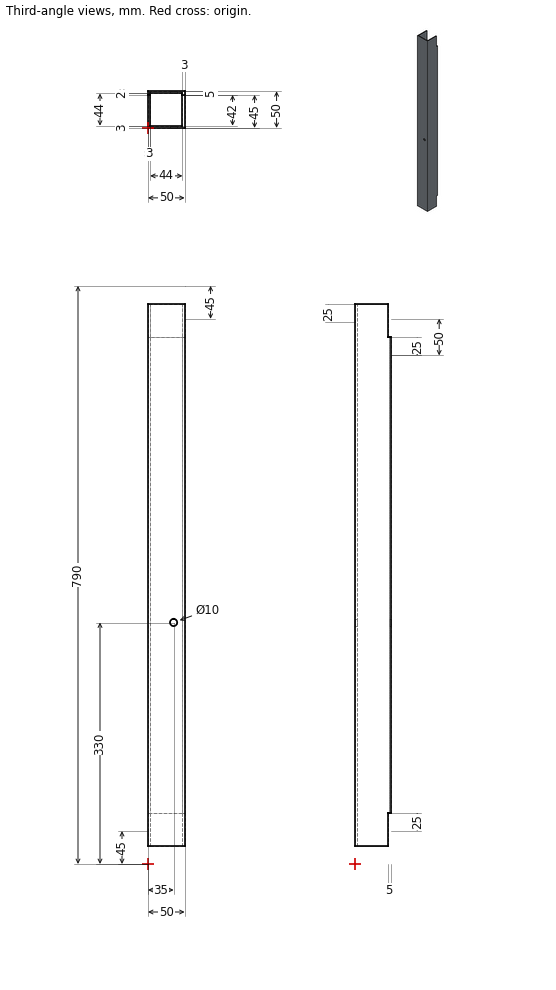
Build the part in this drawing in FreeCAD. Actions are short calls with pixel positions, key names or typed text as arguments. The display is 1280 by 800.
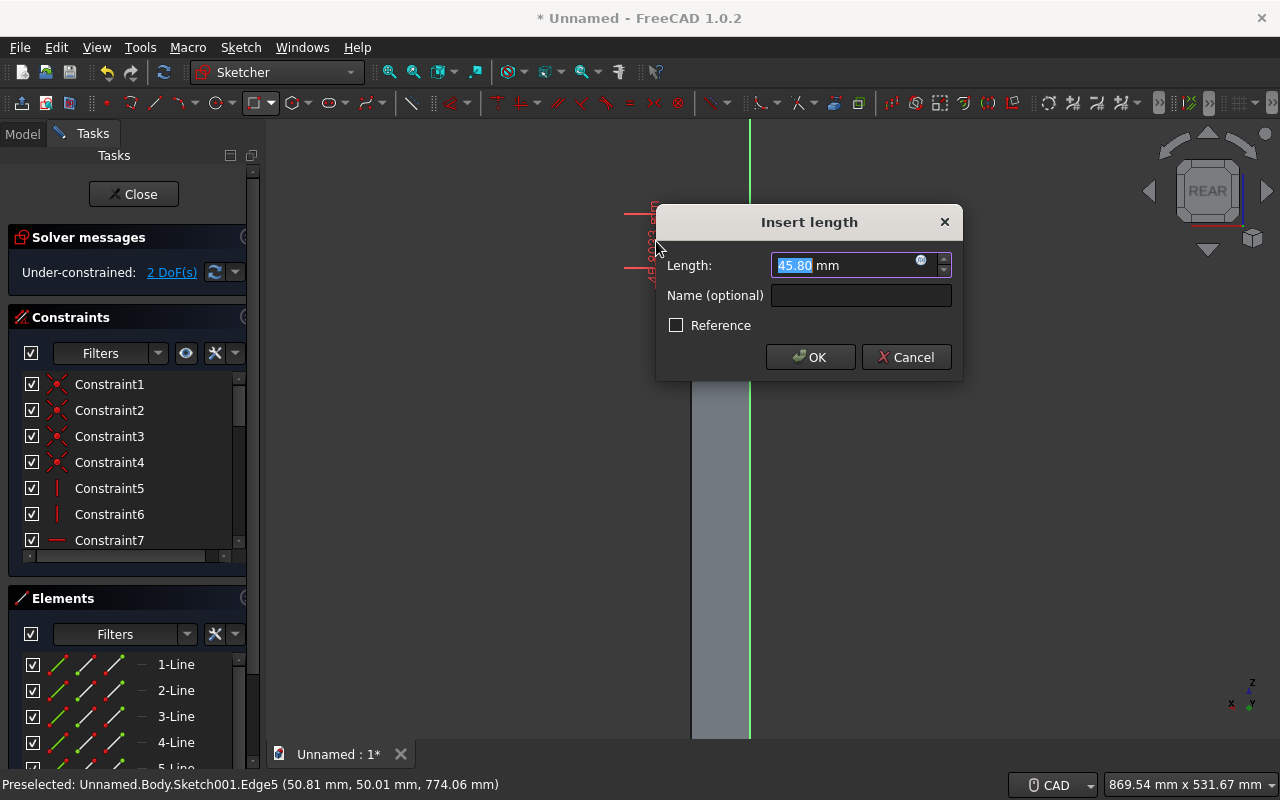
text(45)
key(Return)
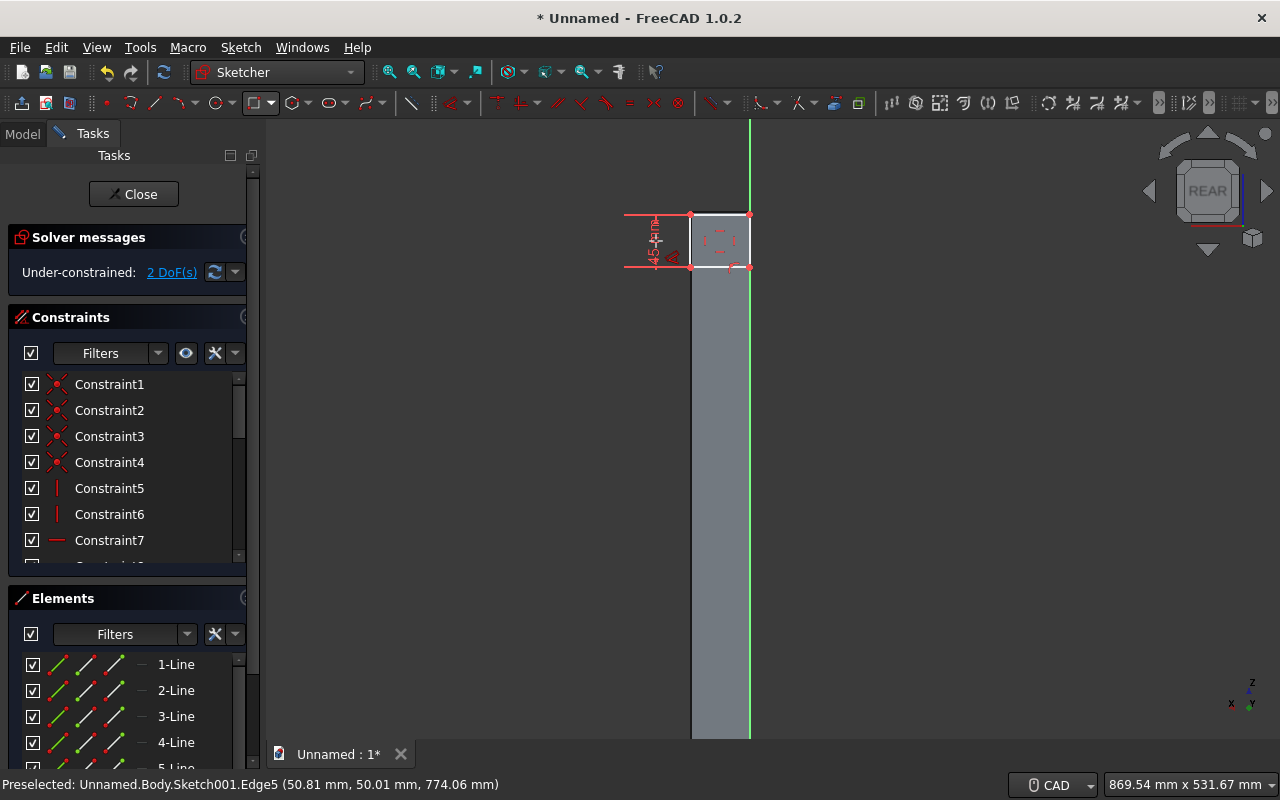
click(708, 267)
click(734, 233)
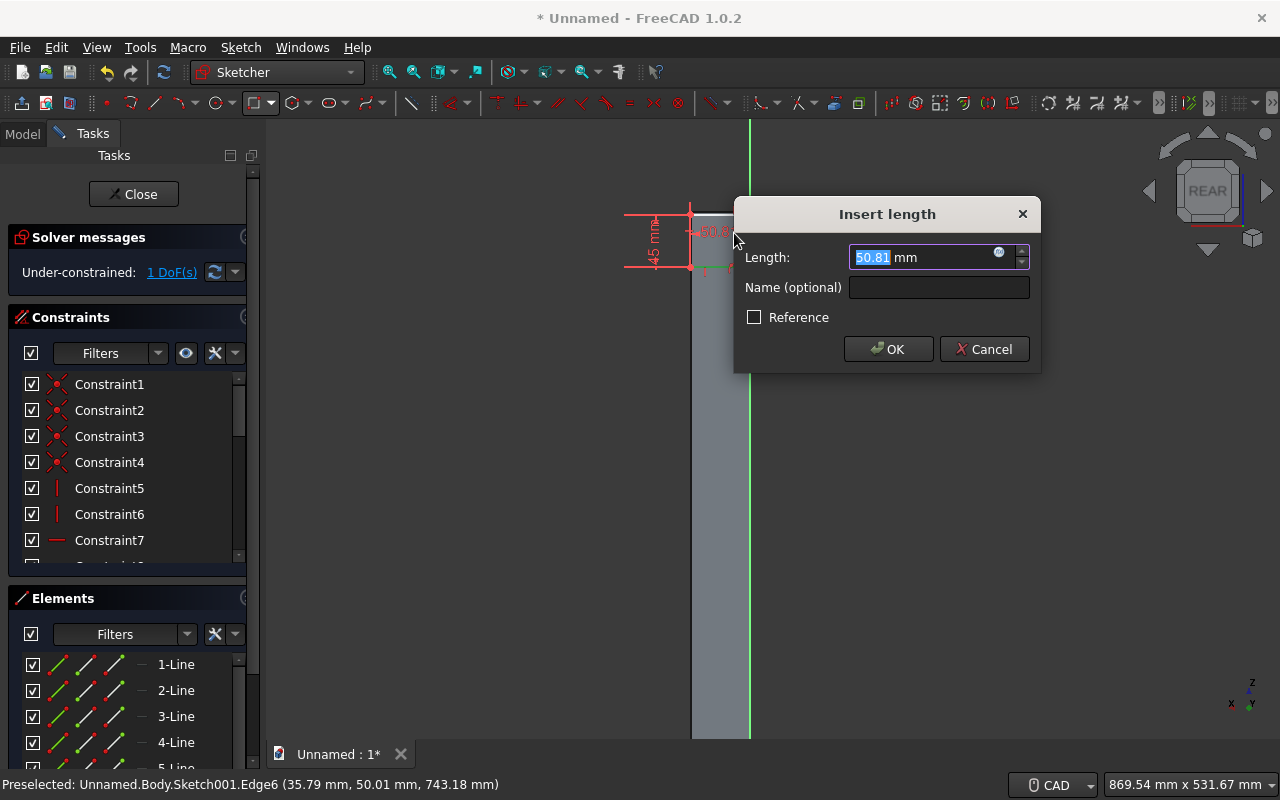
text(50)
key(Return)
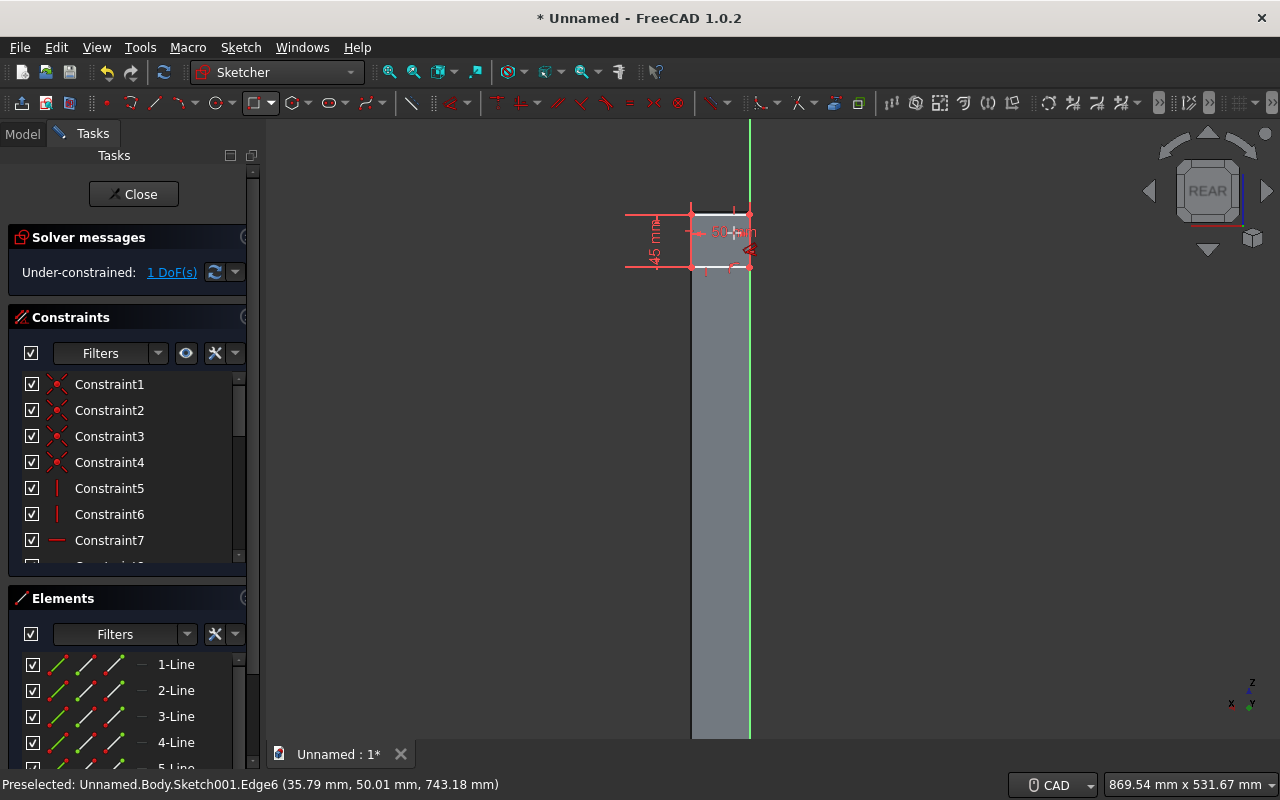
click(691, 215)
click(784, 463)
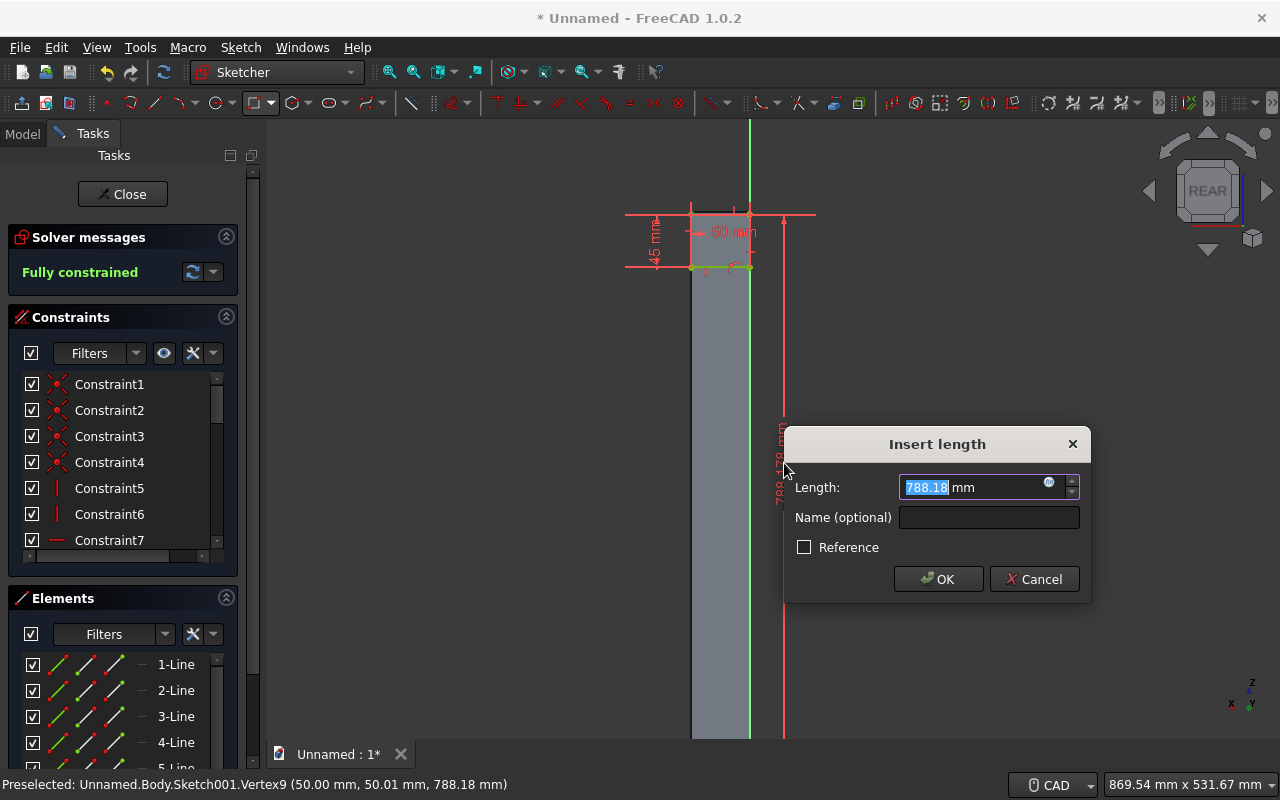
text(790)
key(Return)
key(Escape)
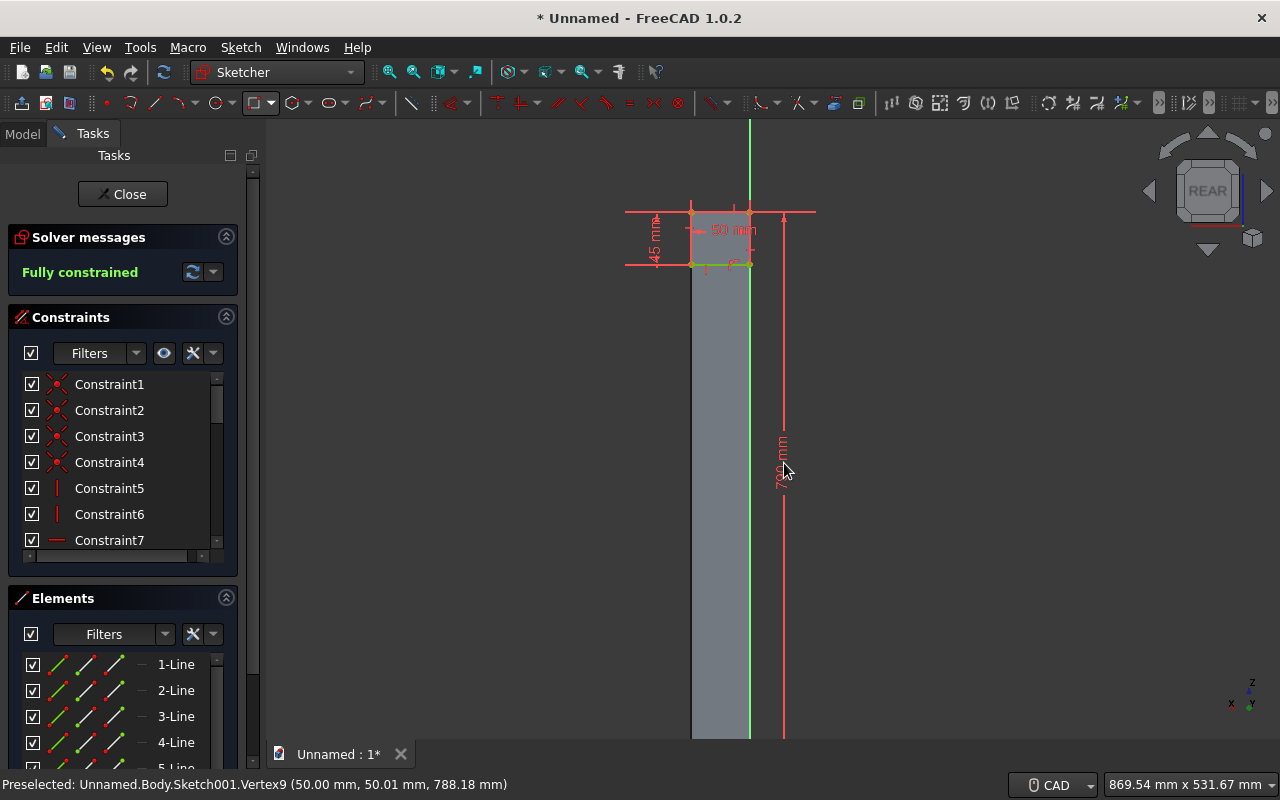
click(123, 194)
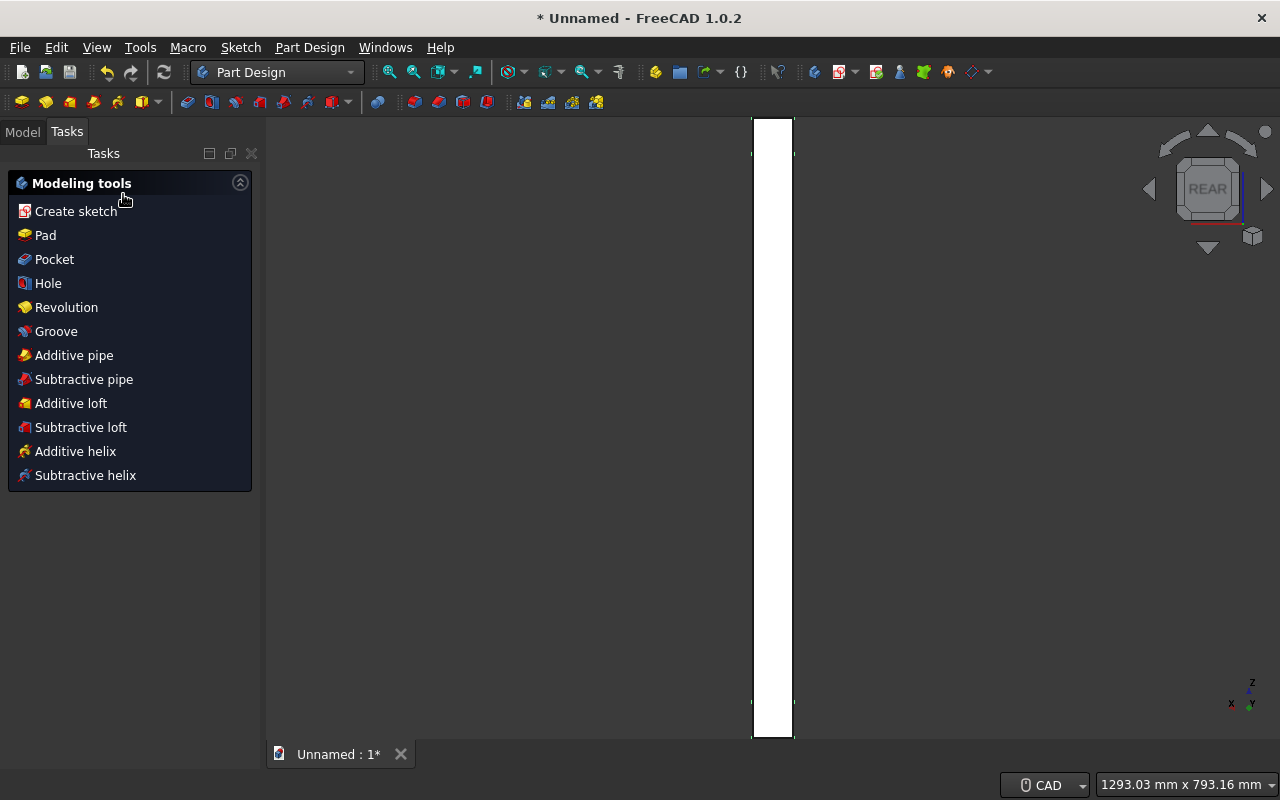
click(188, 102)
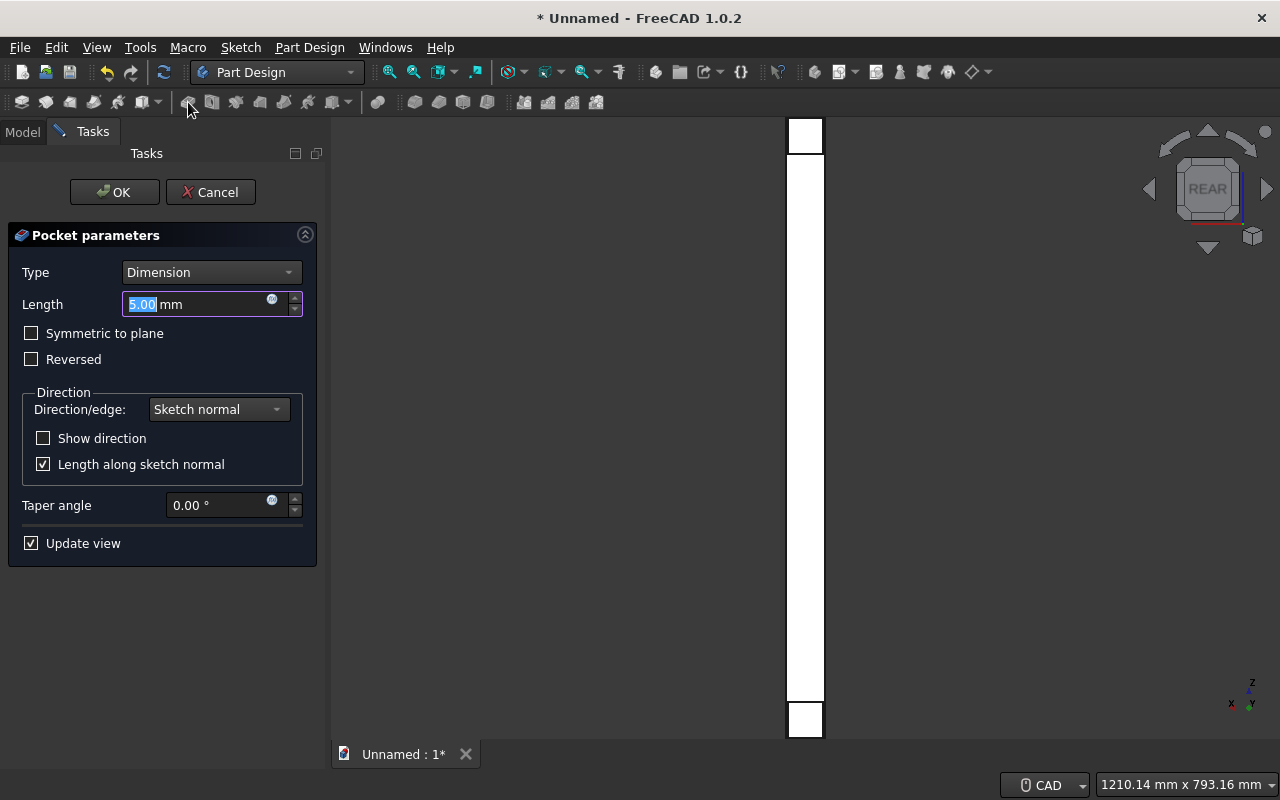
text(5)
key(Tab)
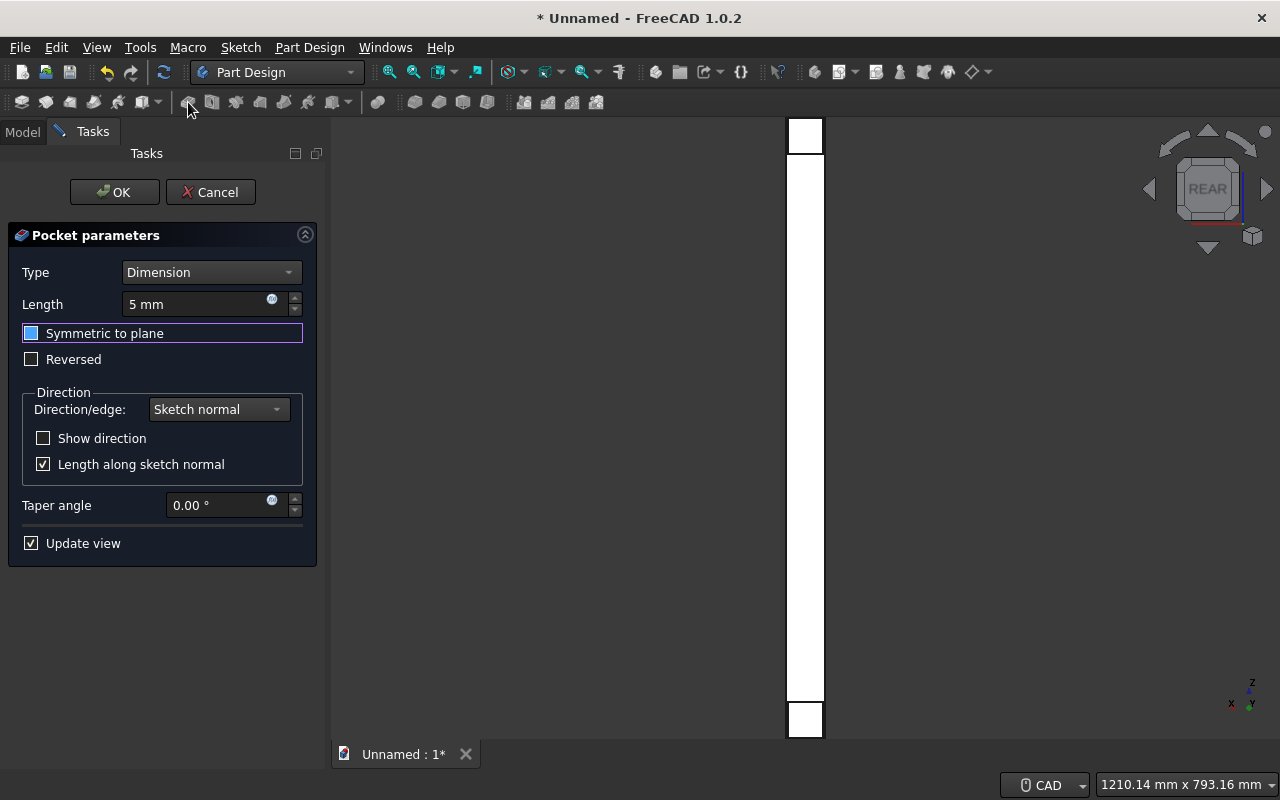
click(115, 192)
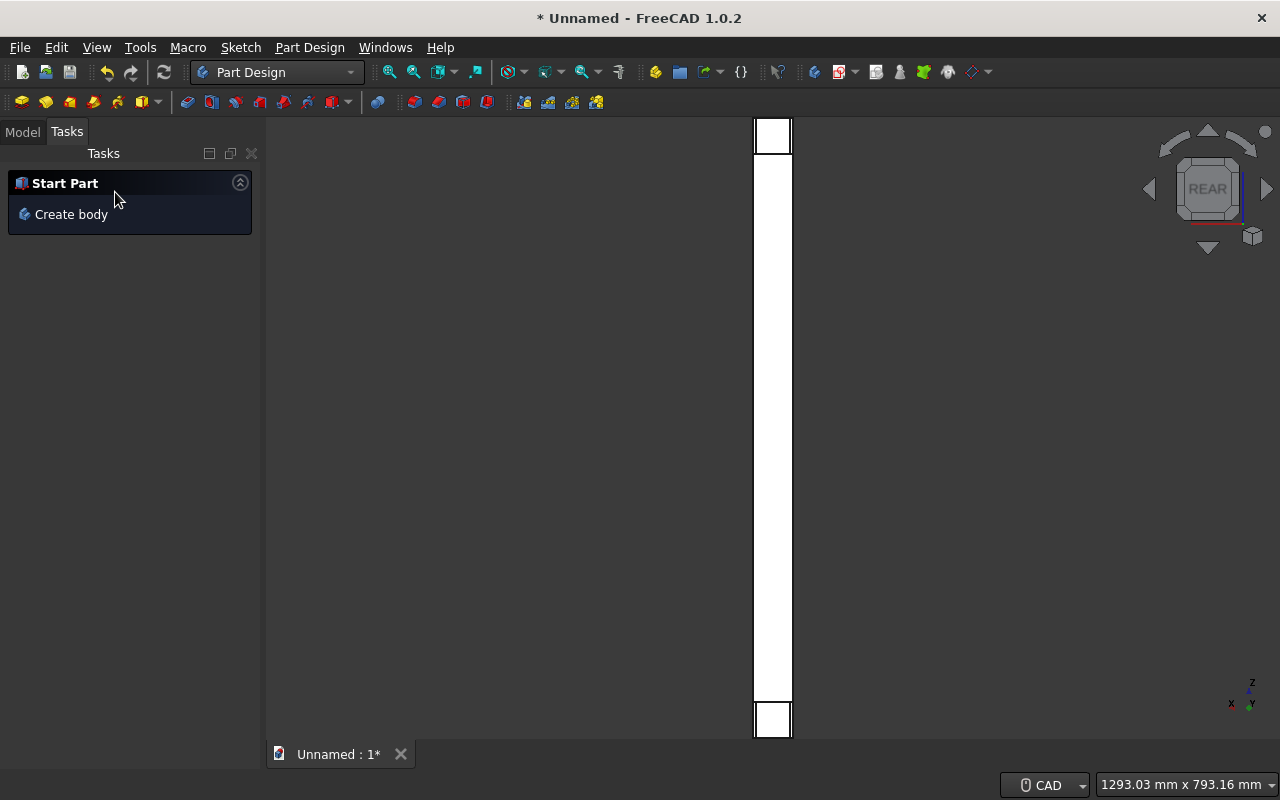
click(773, 192)